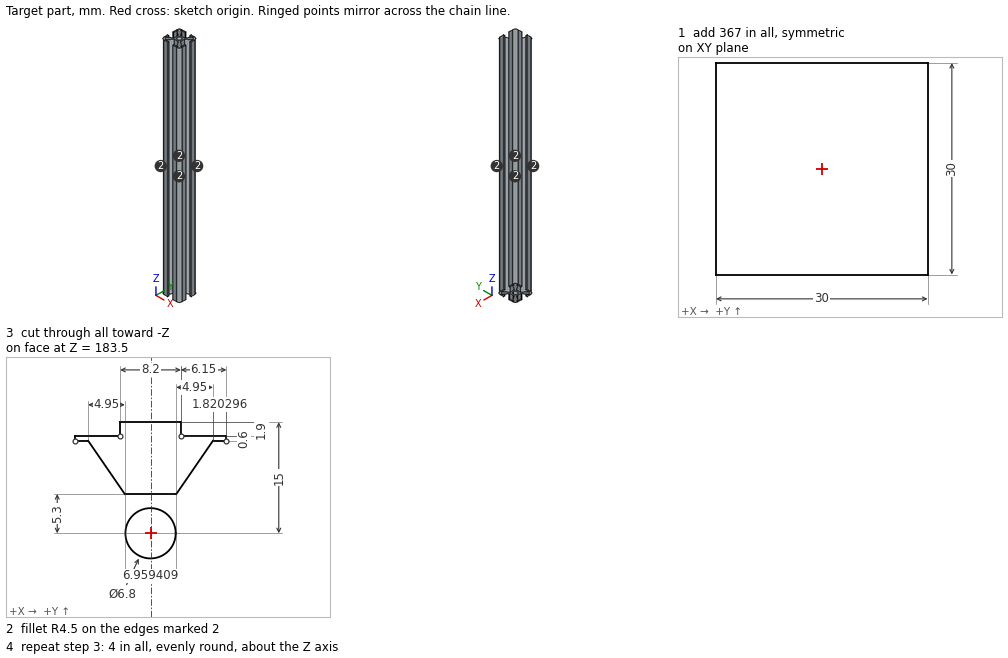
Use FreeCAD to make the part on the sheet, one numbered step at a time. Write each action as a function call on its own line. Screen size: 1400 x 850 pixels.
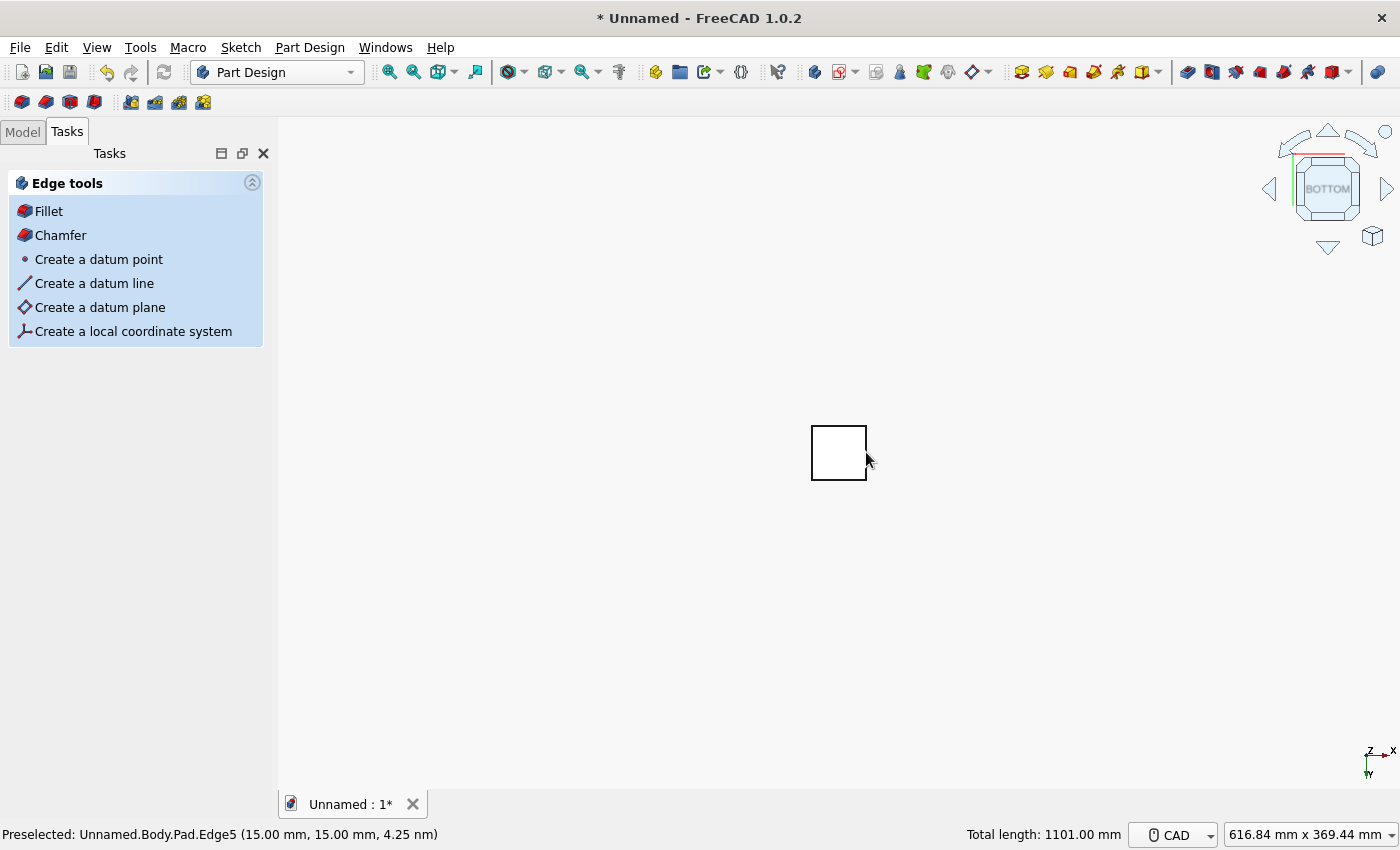
key(v)
key(f)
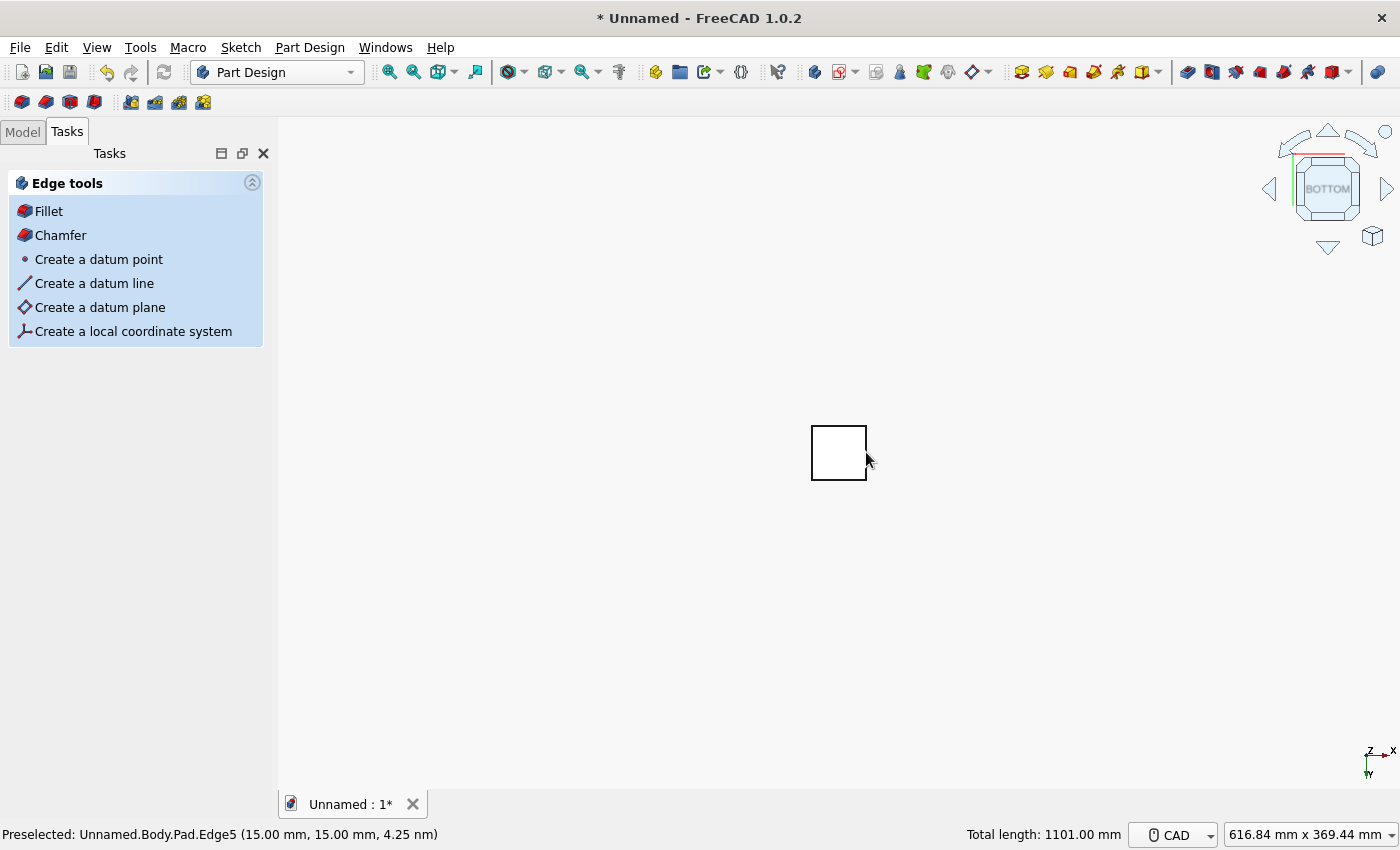
key(4)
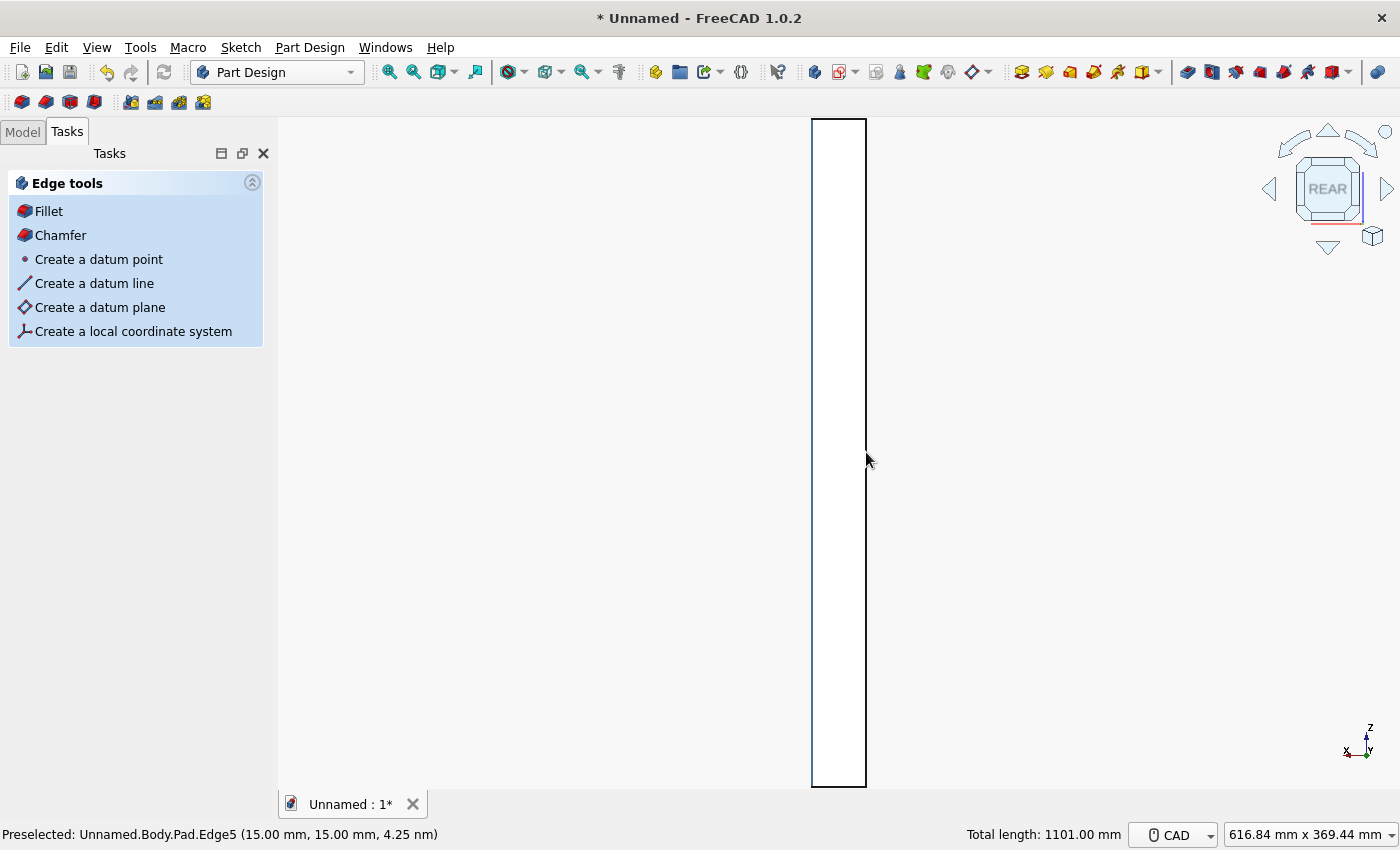
click(866, 452, ctrl)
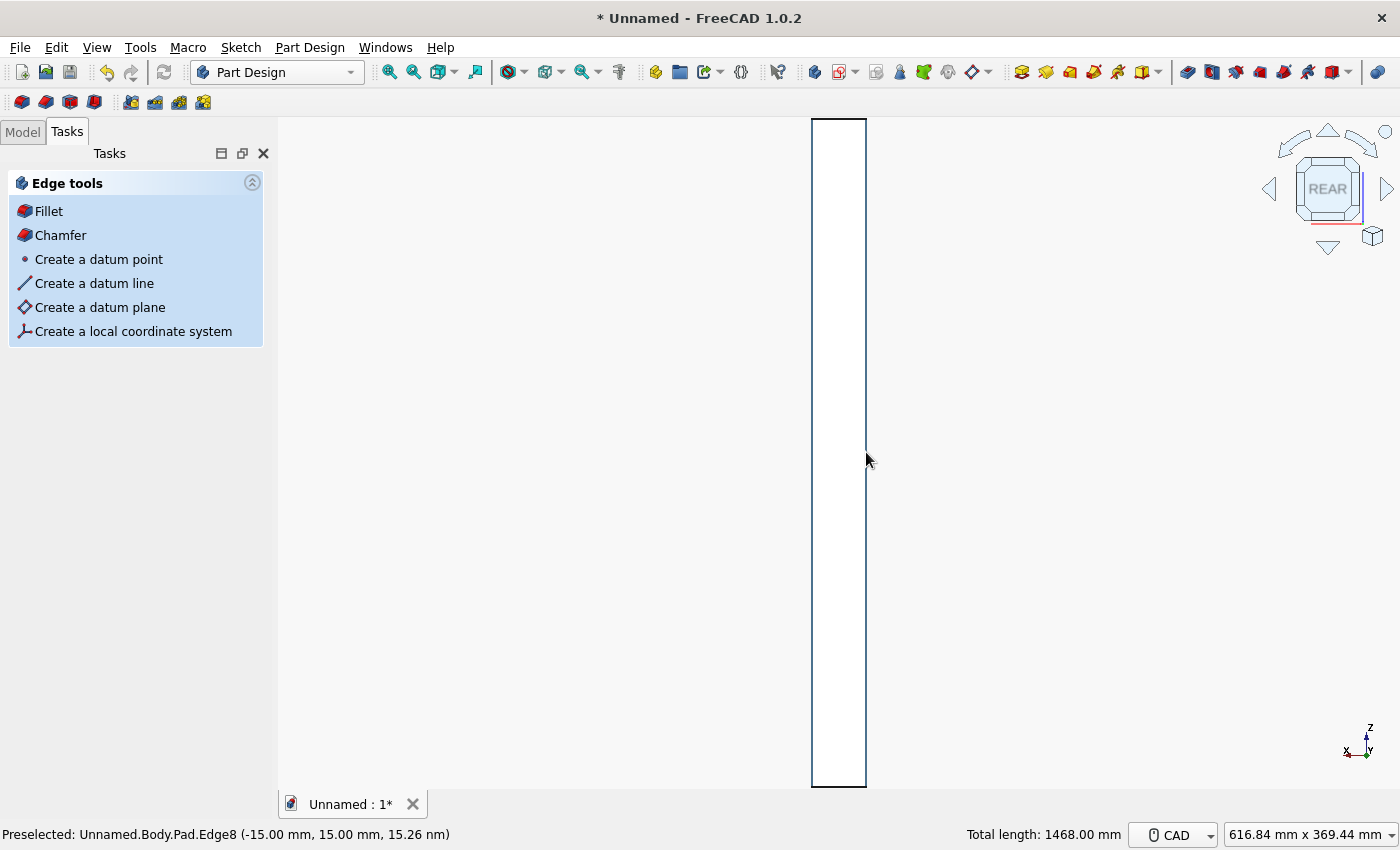
click(22, 102)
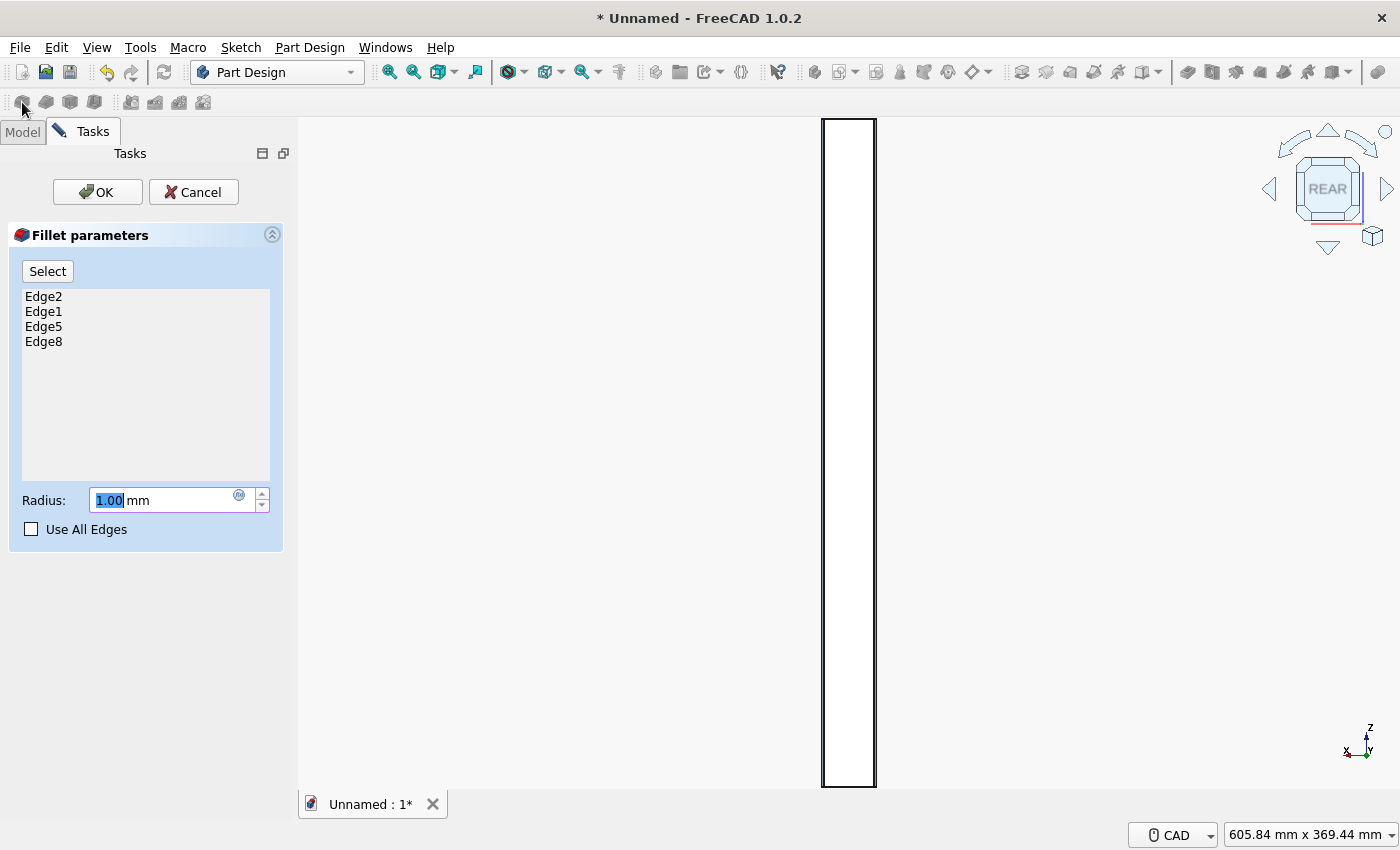
text(4.5)
key(Tab)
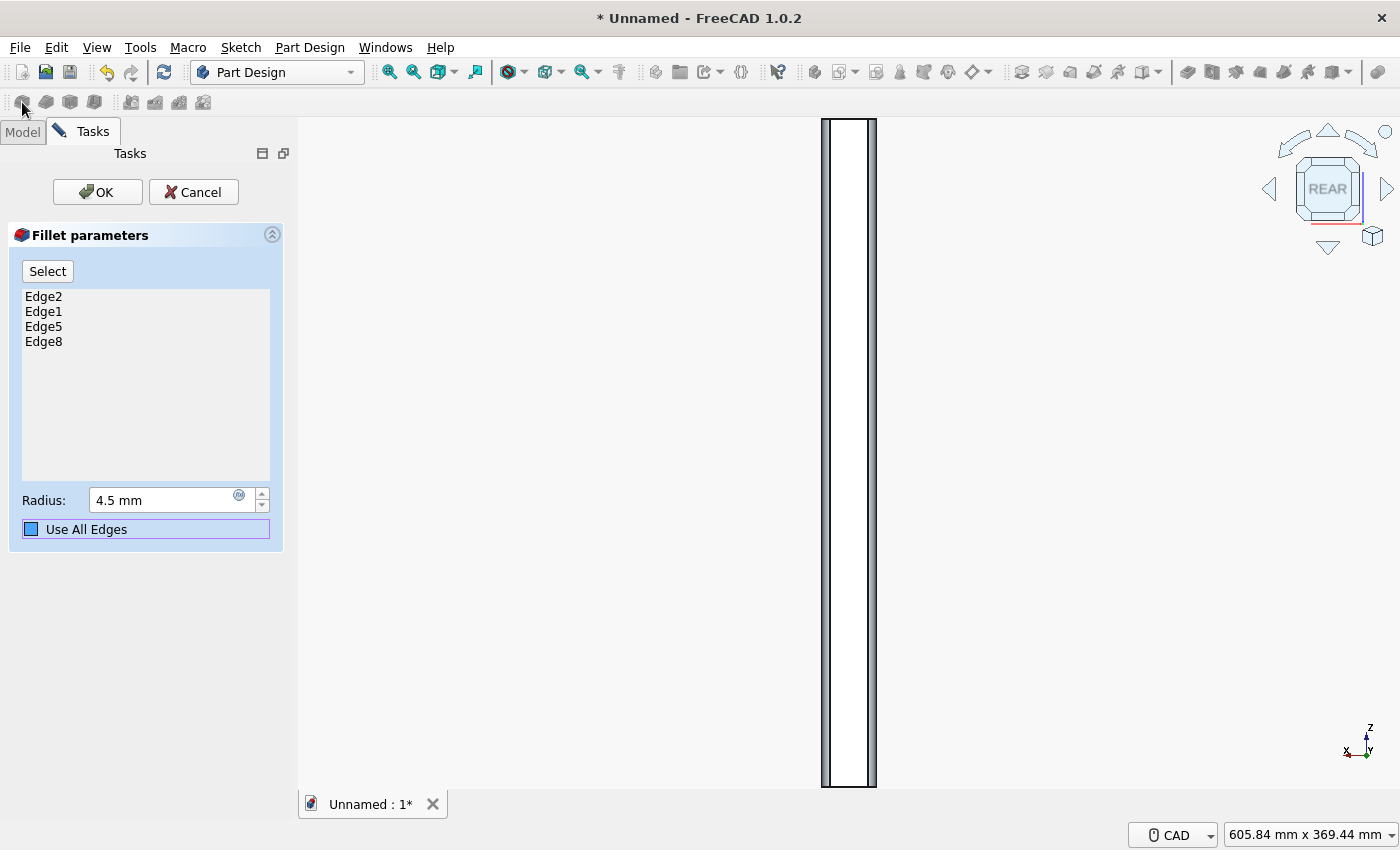
click(98, 192)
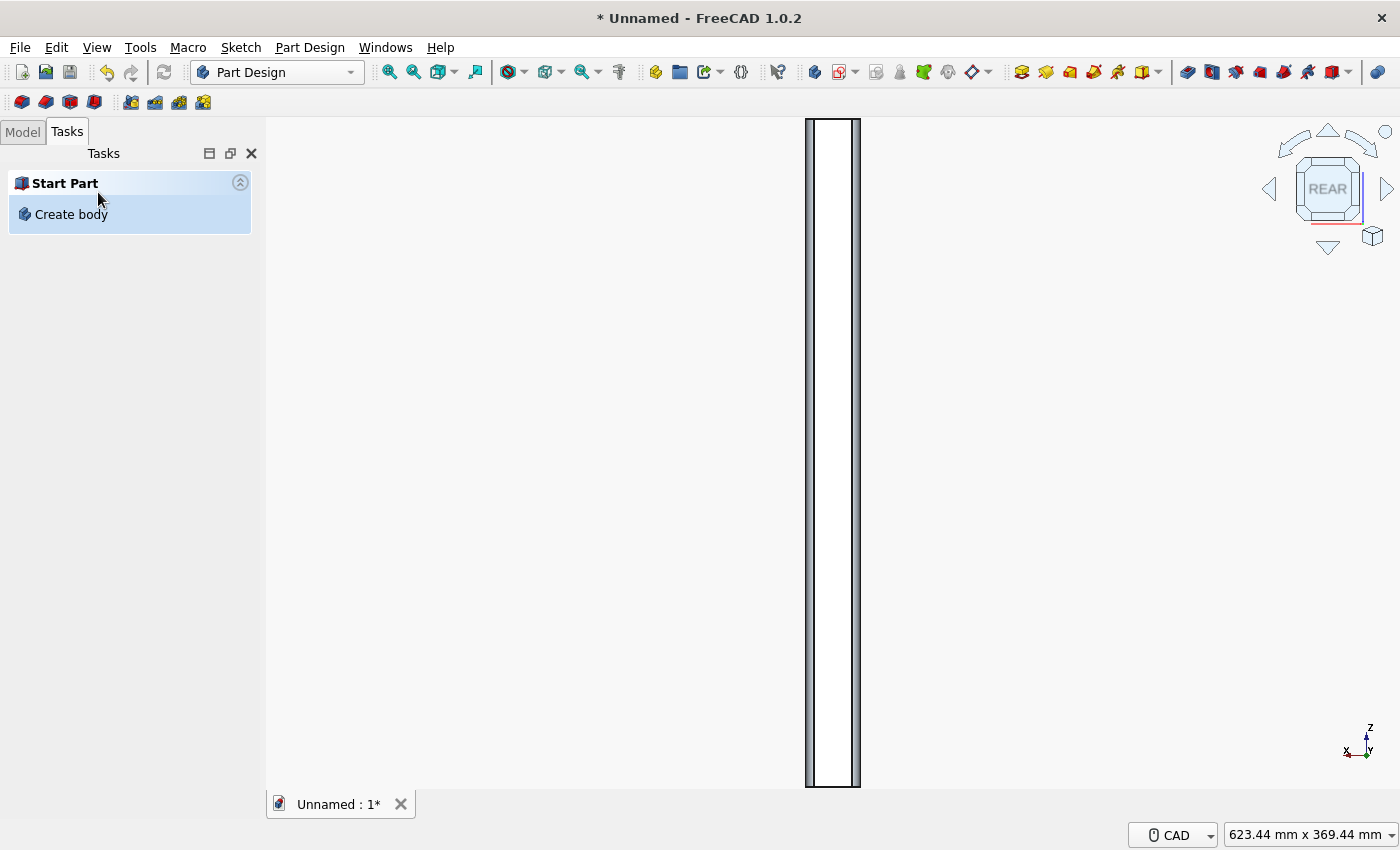
key(0)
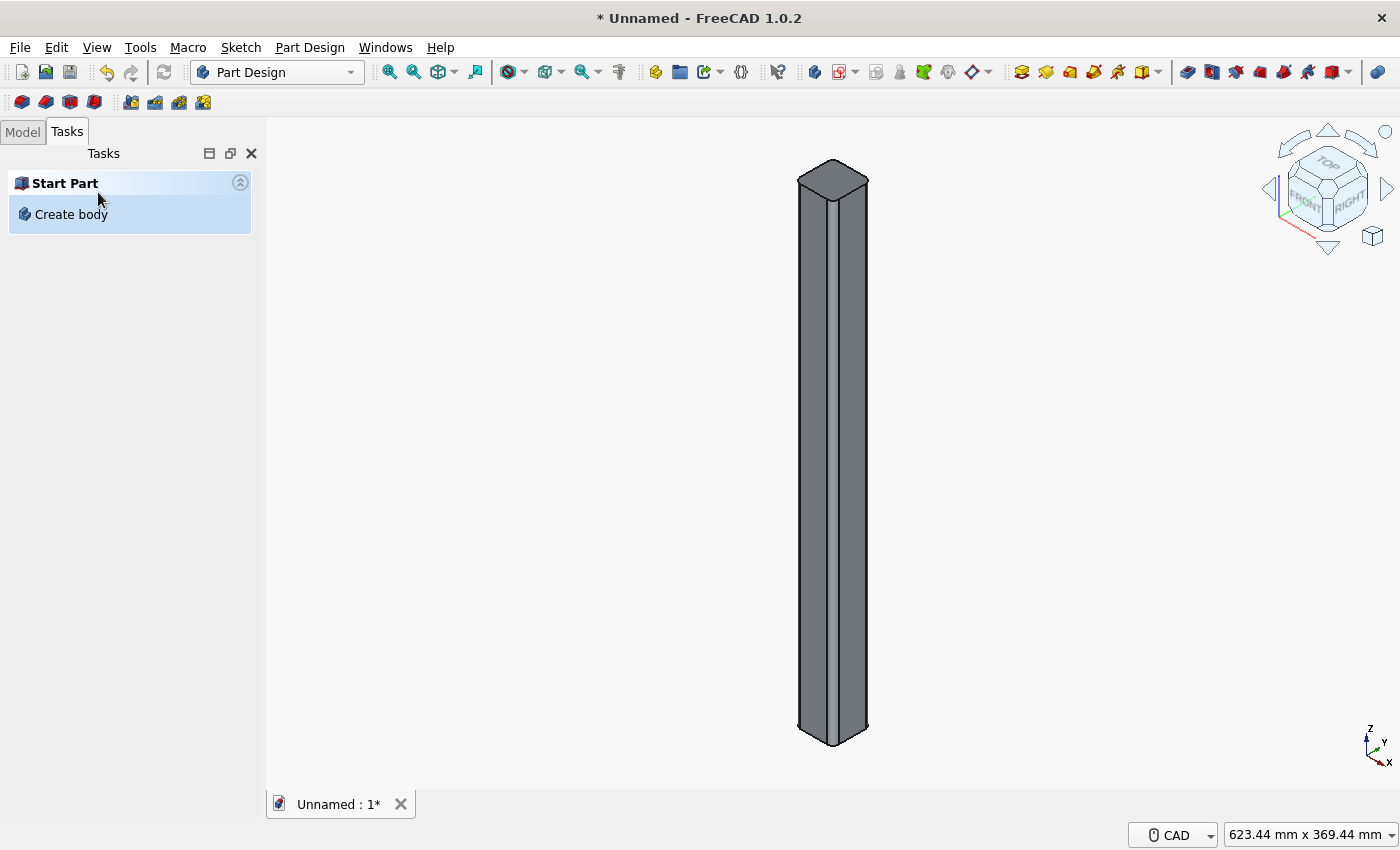
click(833, 179)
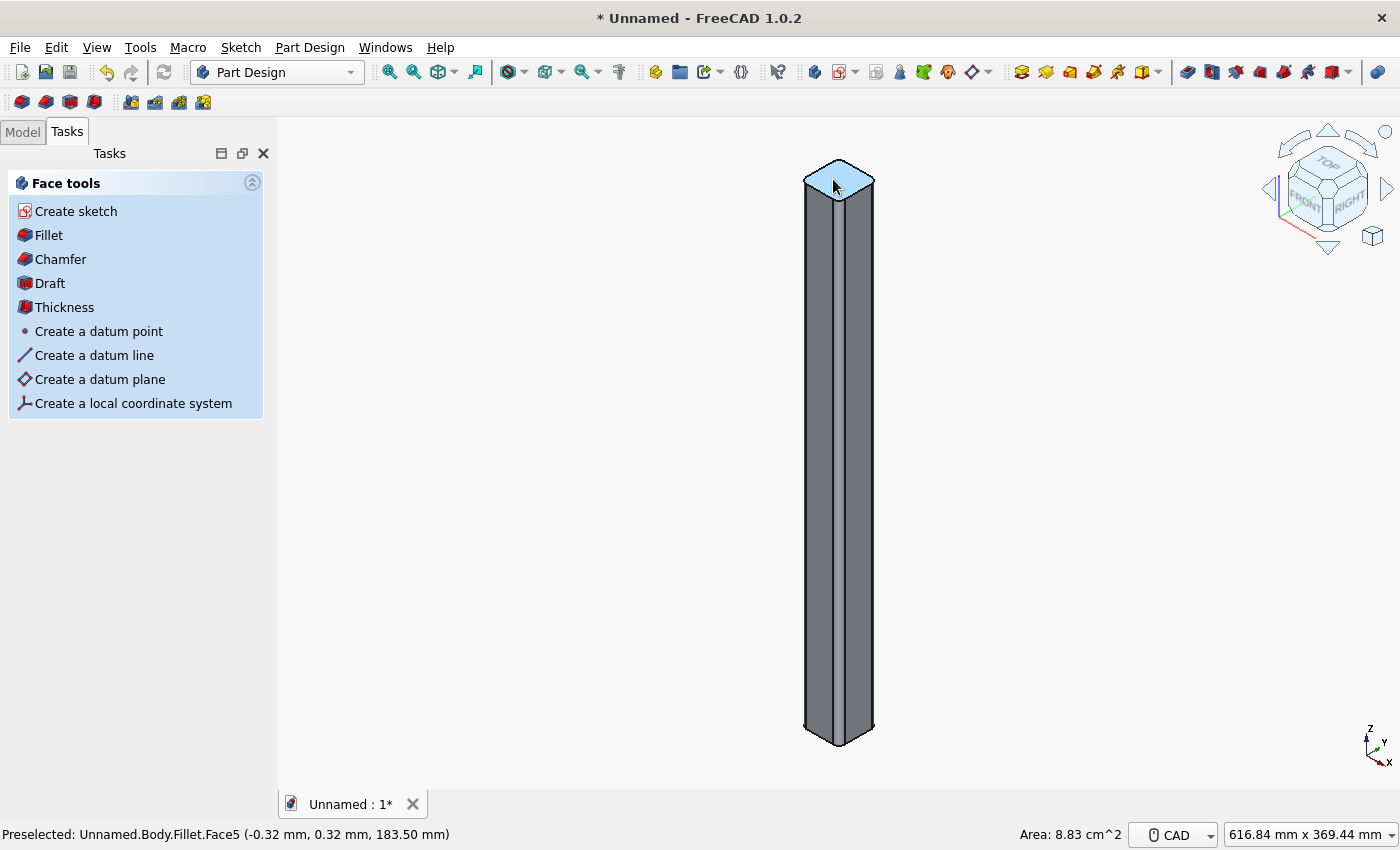
click(840, 72)